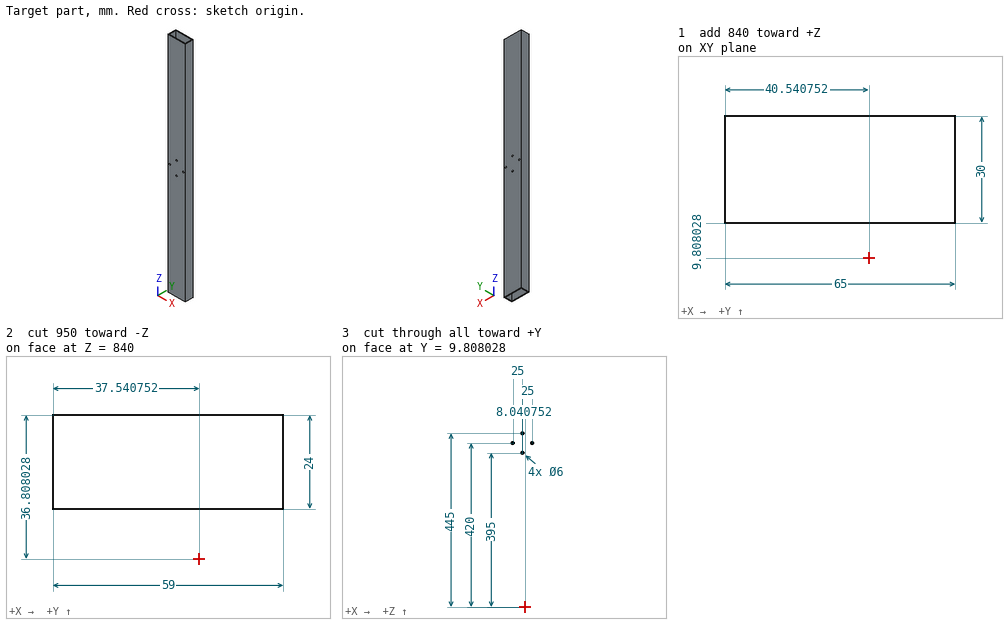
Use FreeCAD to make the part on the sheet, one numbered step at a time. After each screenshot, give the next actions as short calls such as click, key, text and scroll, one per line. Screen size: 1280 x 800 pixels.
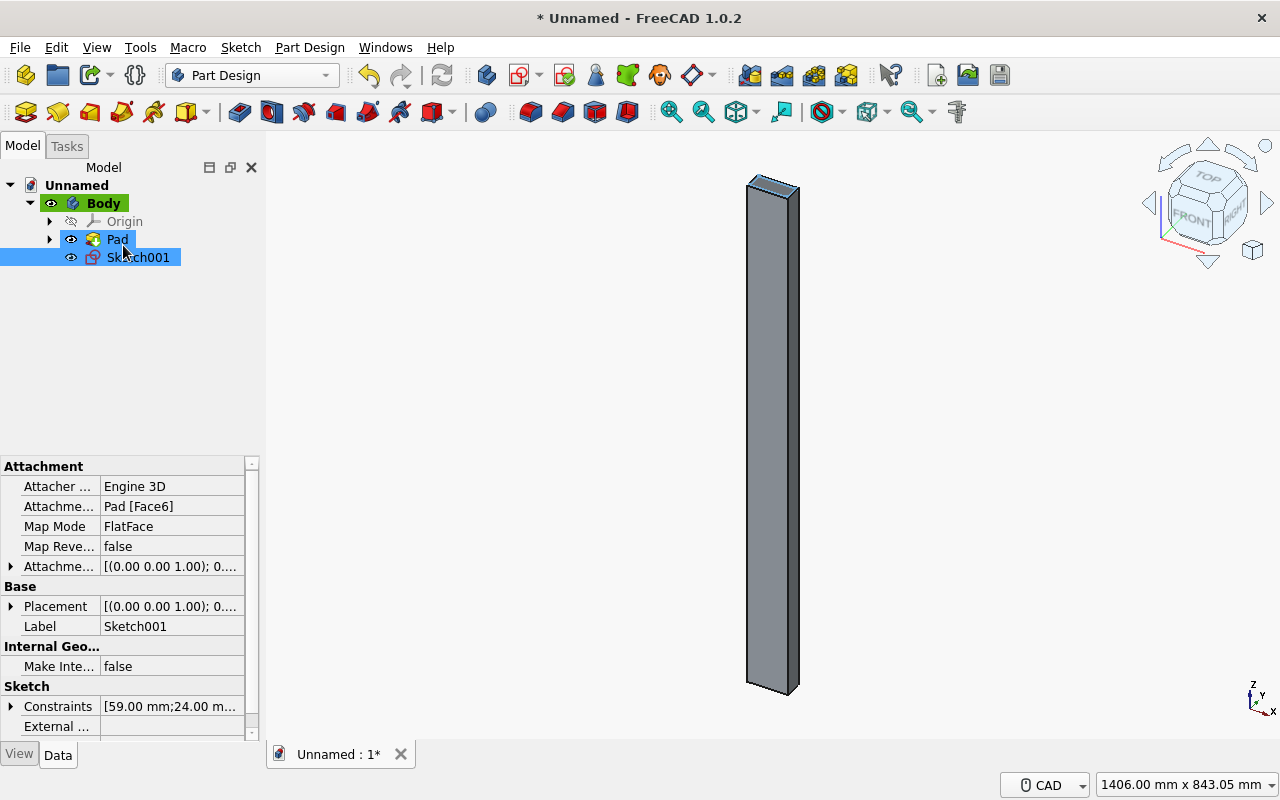
click(240, 112)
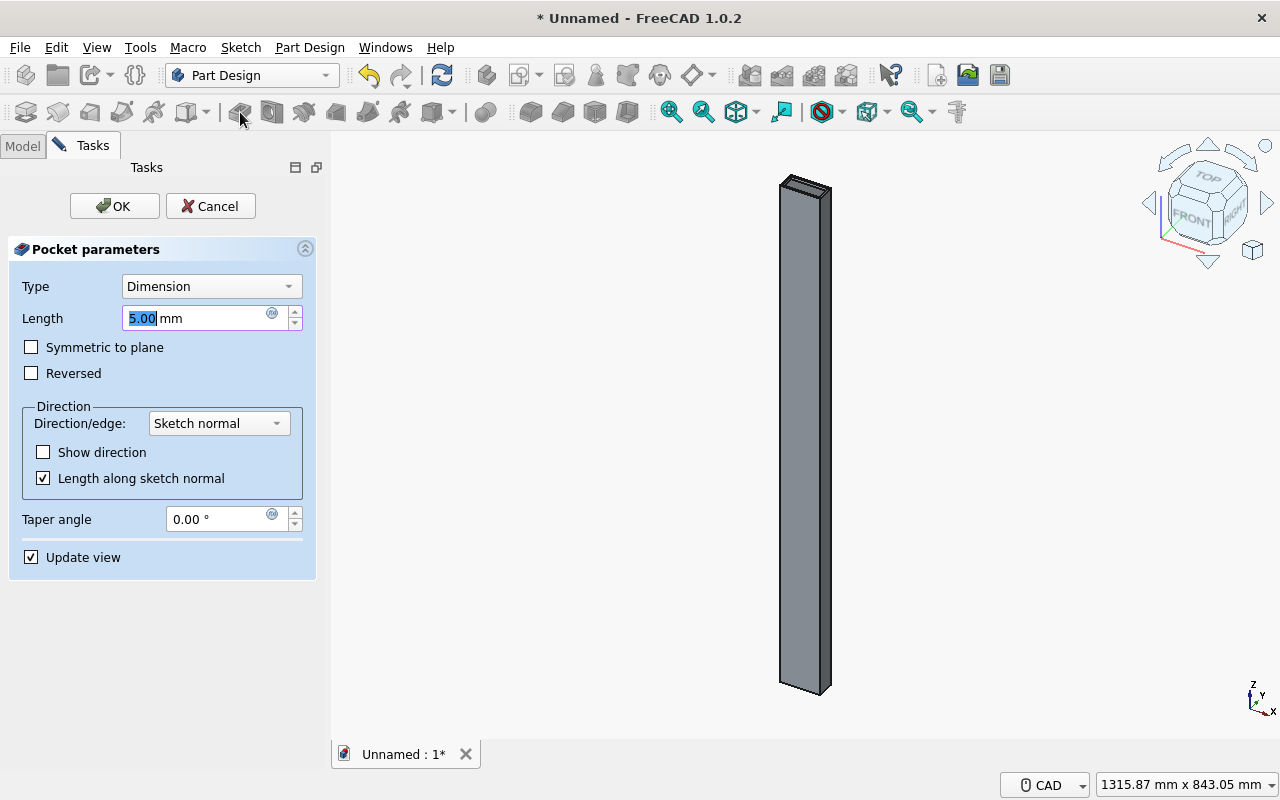
text(950)
key(Tab)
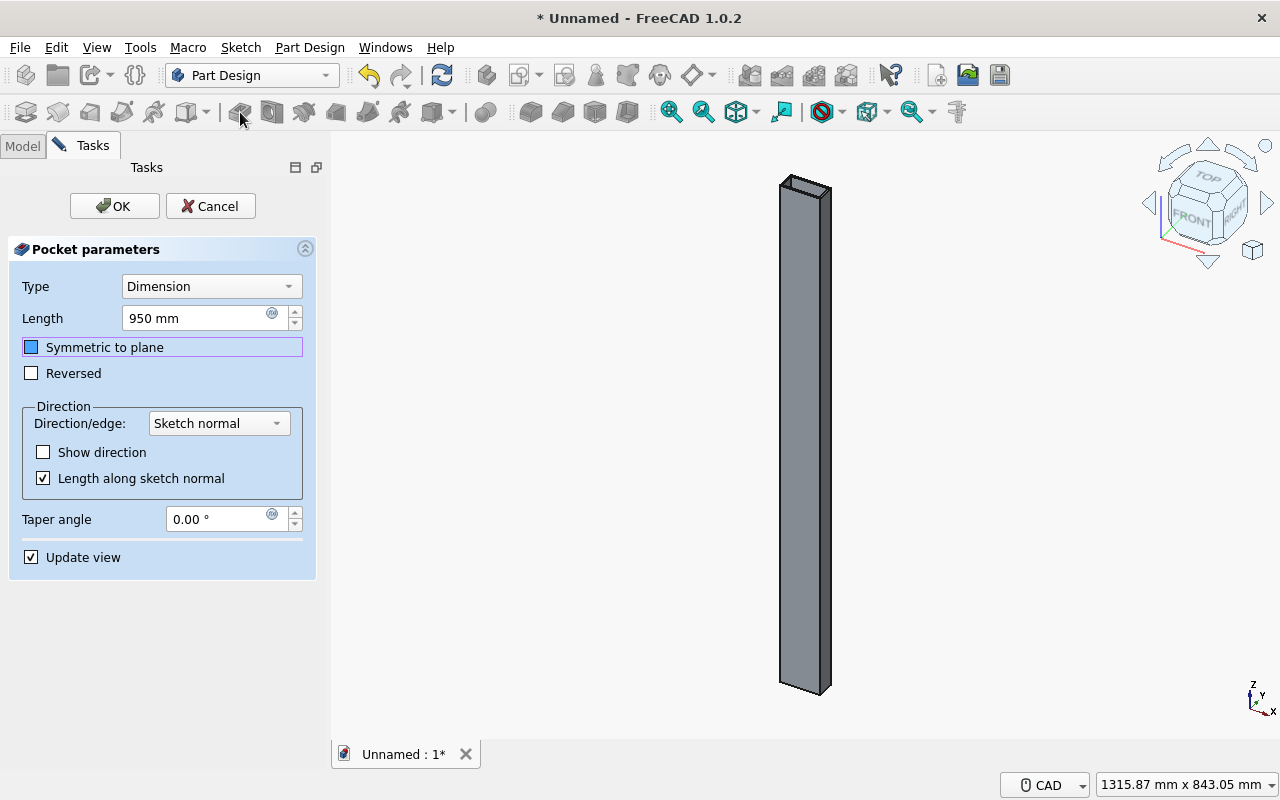
click(115, 206)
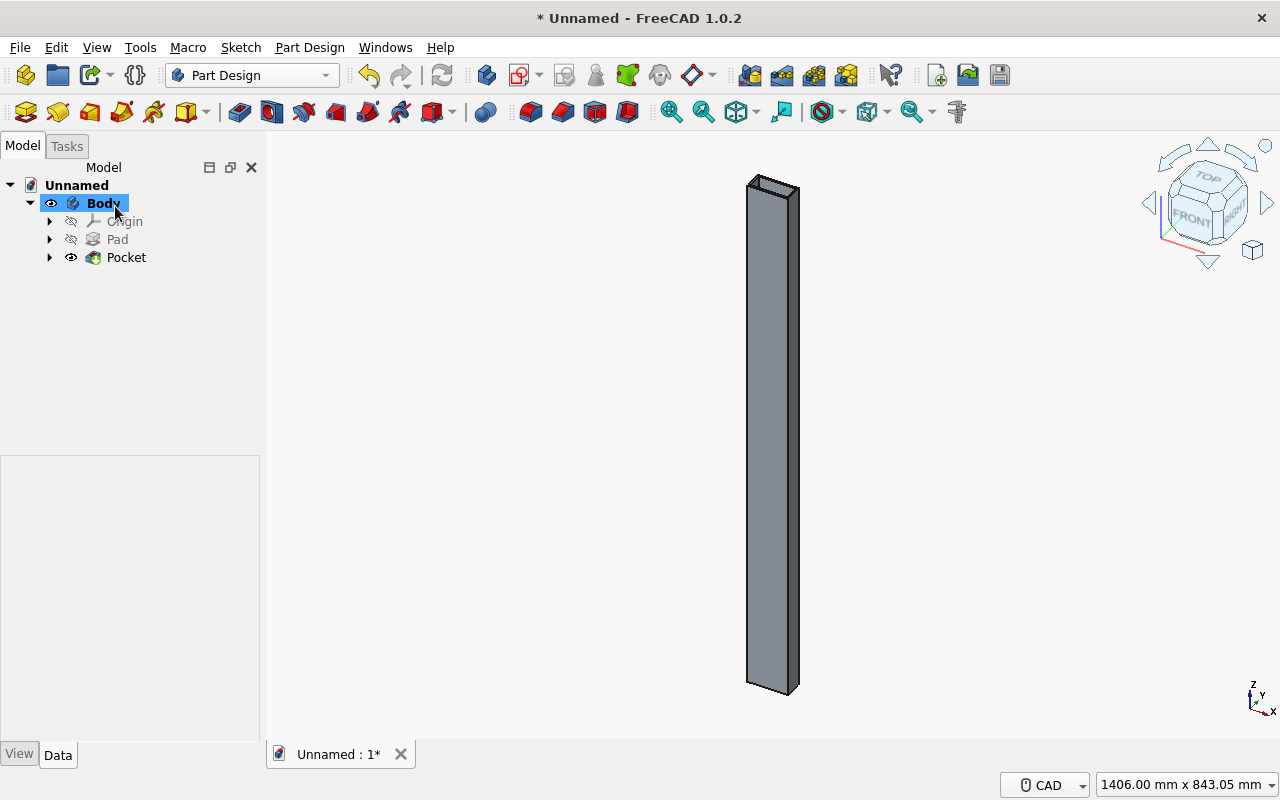
click(768, 227)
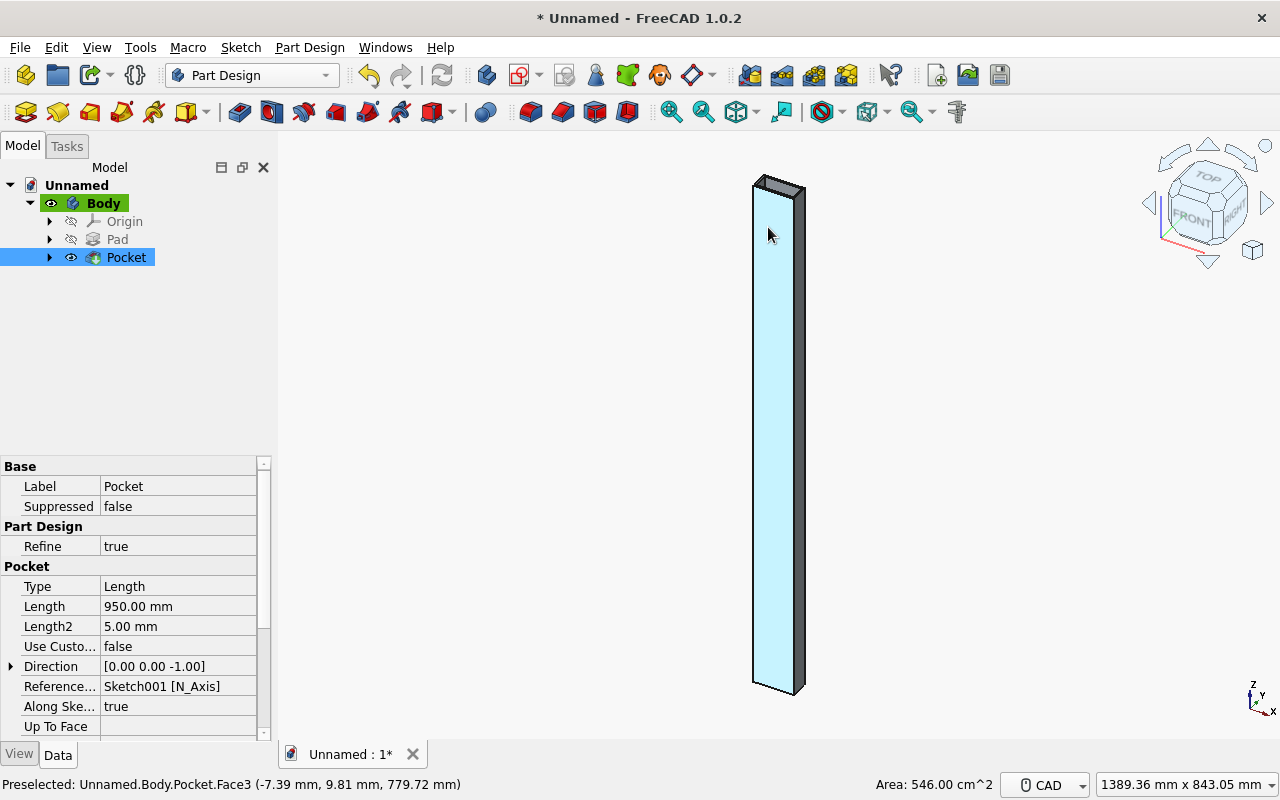
click(520, 76)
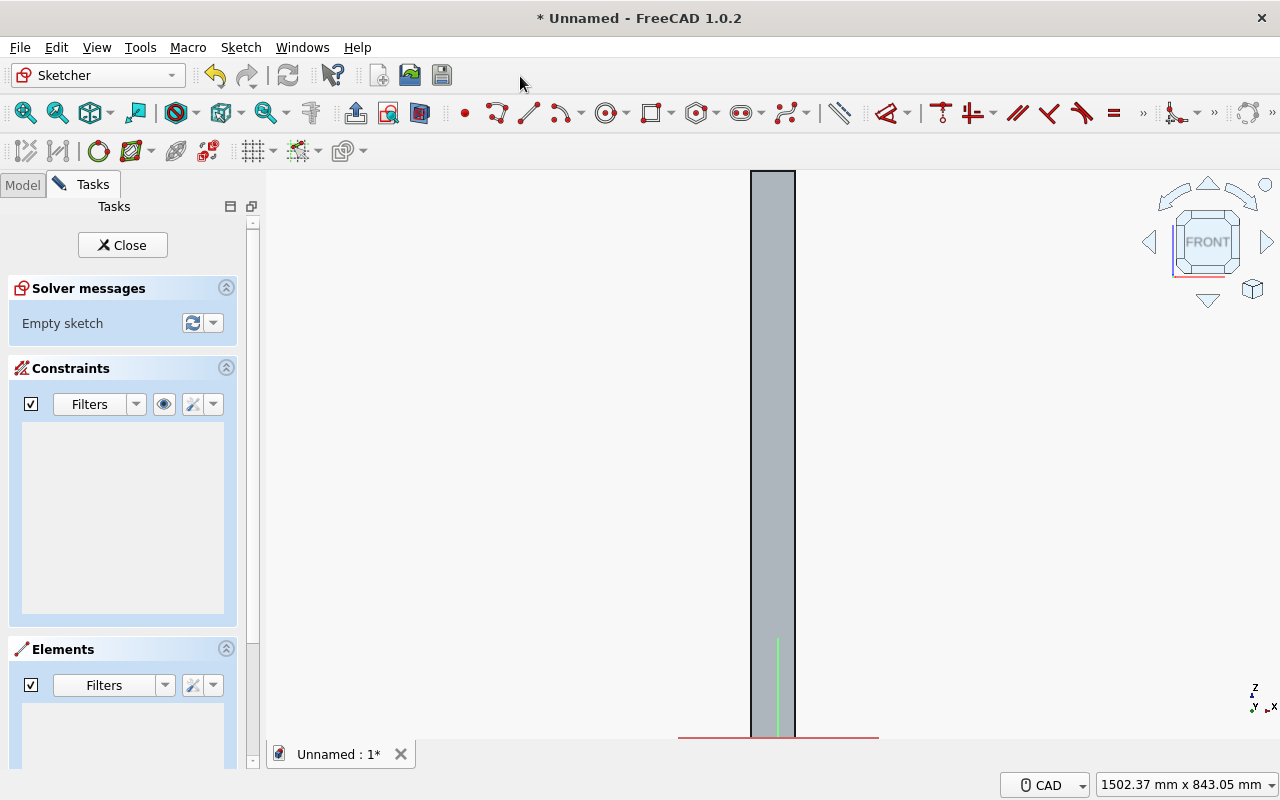
scroll(782, 454, up, 11)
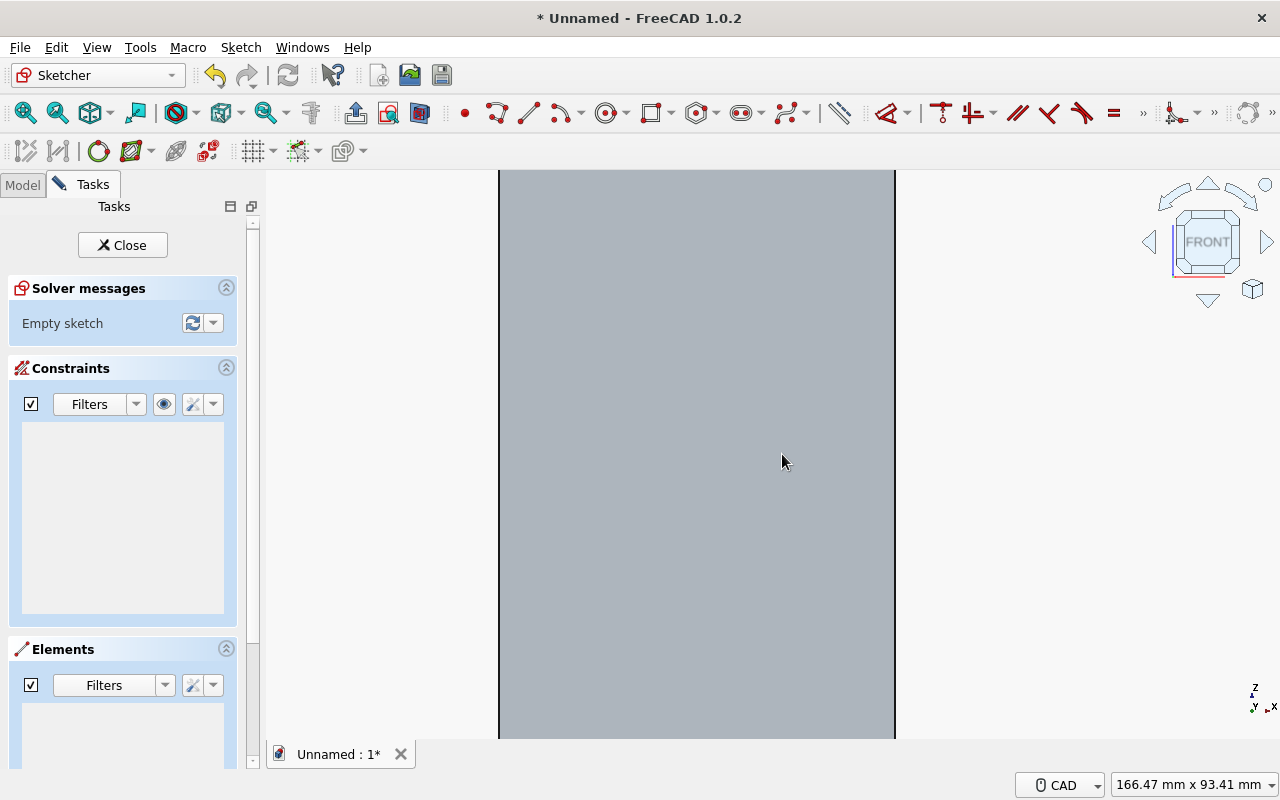
click(606, 114)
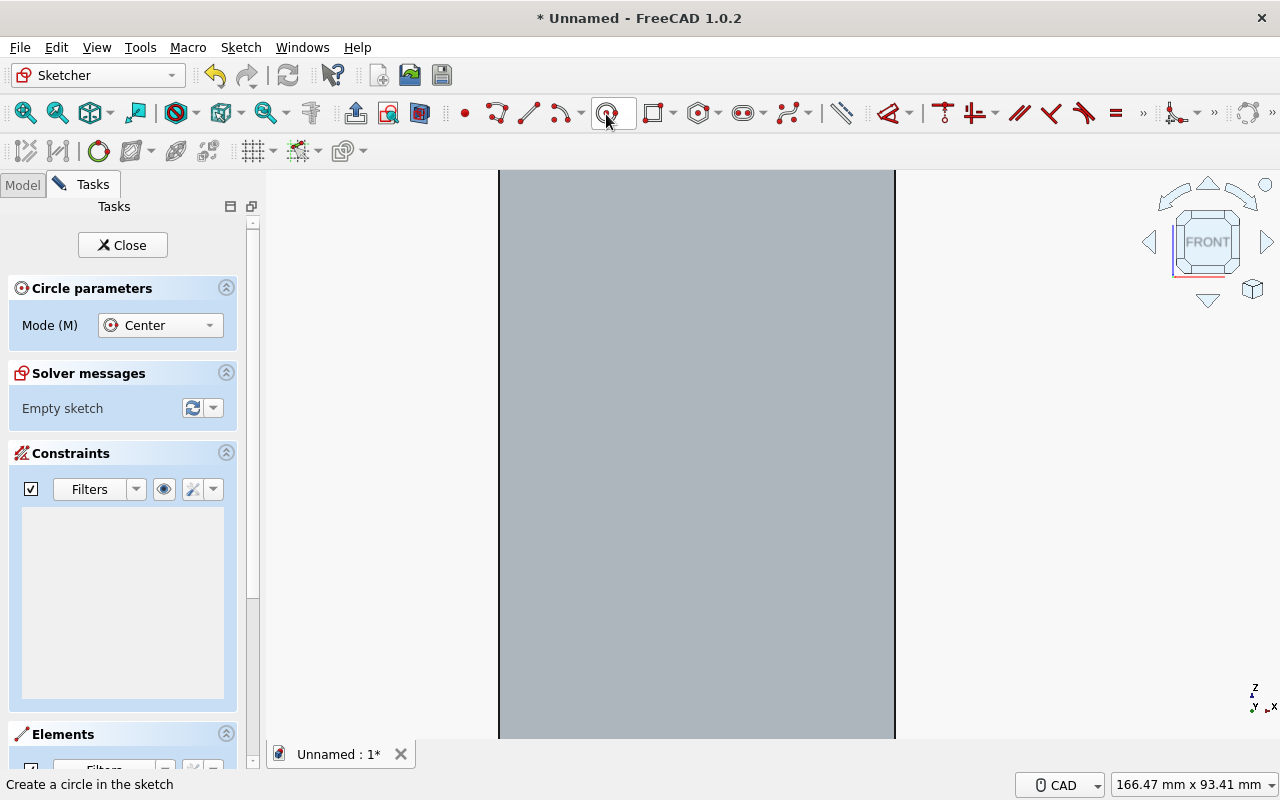
scroll(697, 607, up, 2)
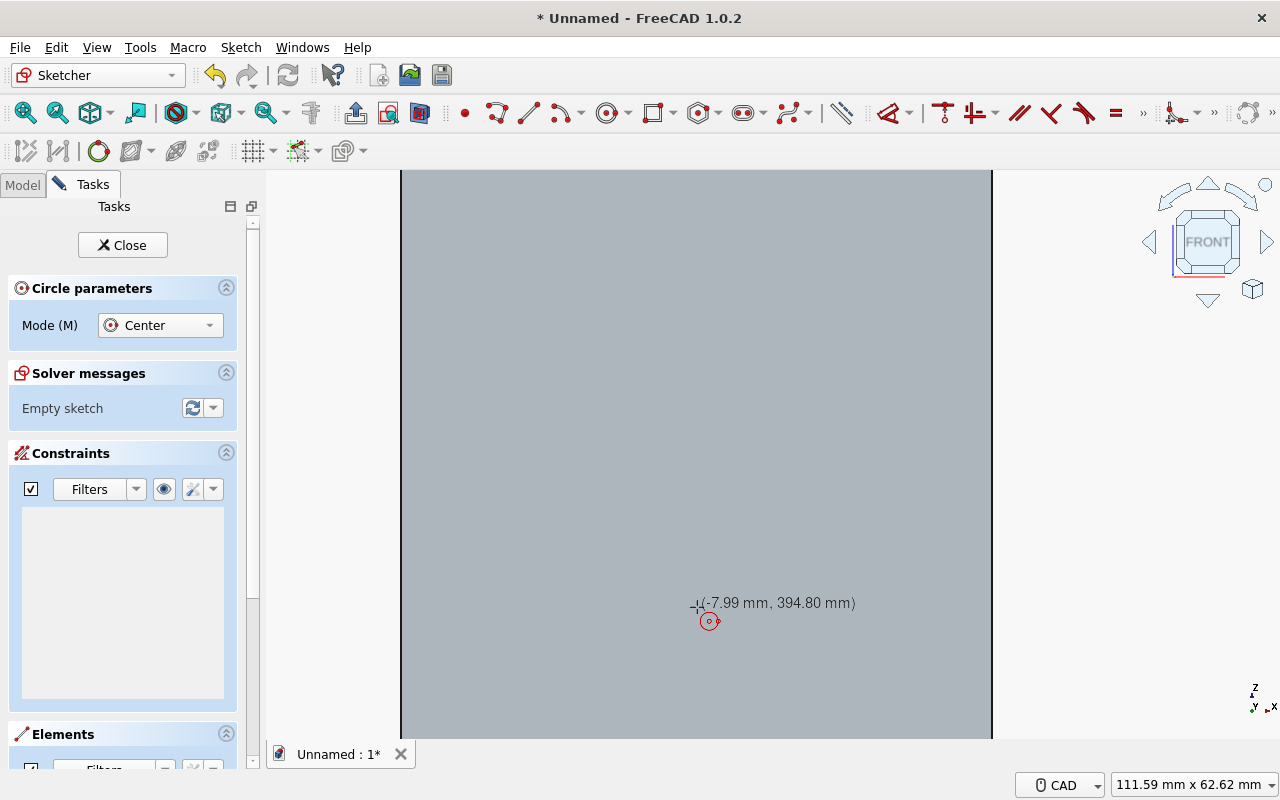
click(696, 606)
move(716, 587)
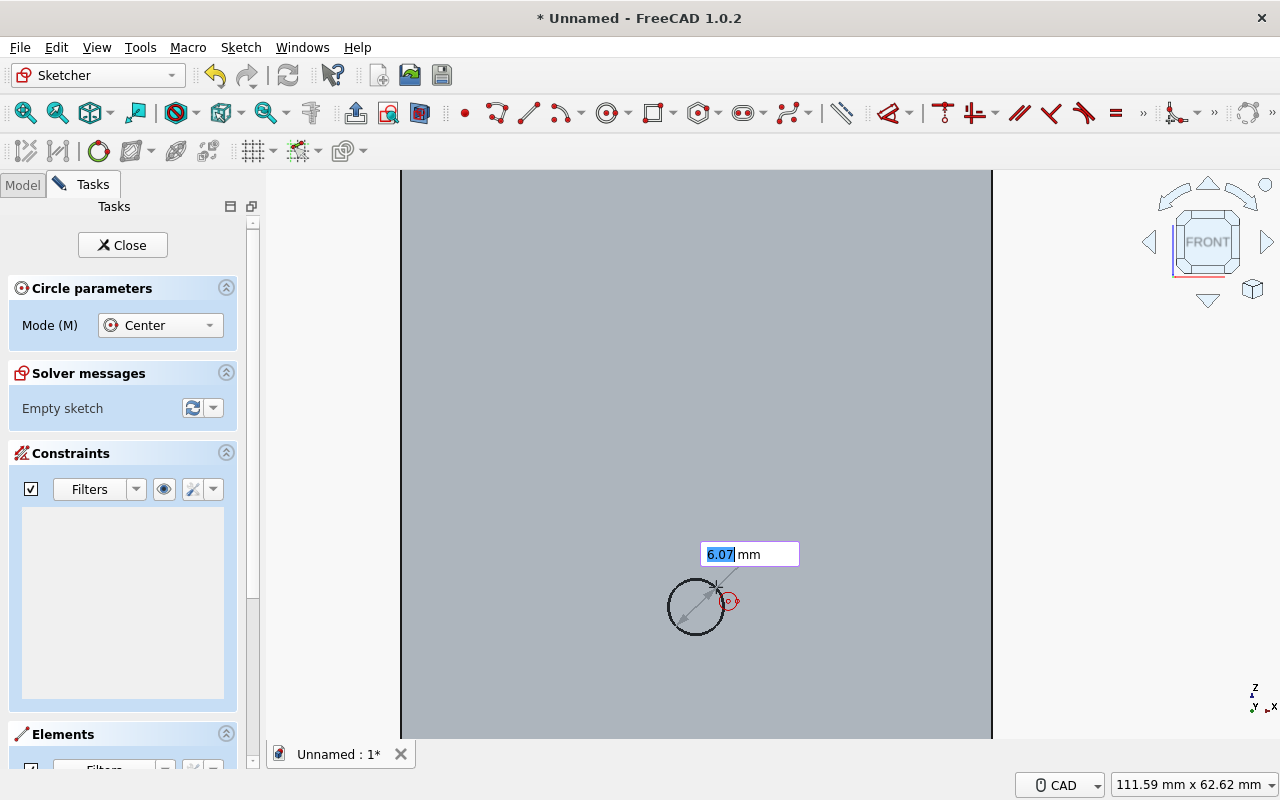
text(6)
key(Return)